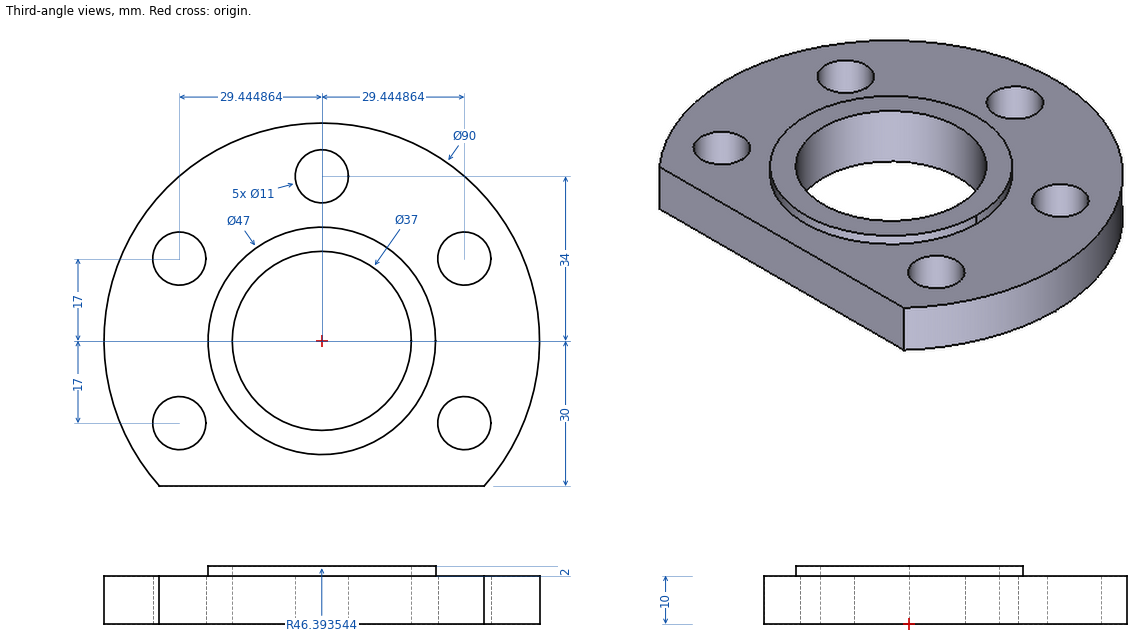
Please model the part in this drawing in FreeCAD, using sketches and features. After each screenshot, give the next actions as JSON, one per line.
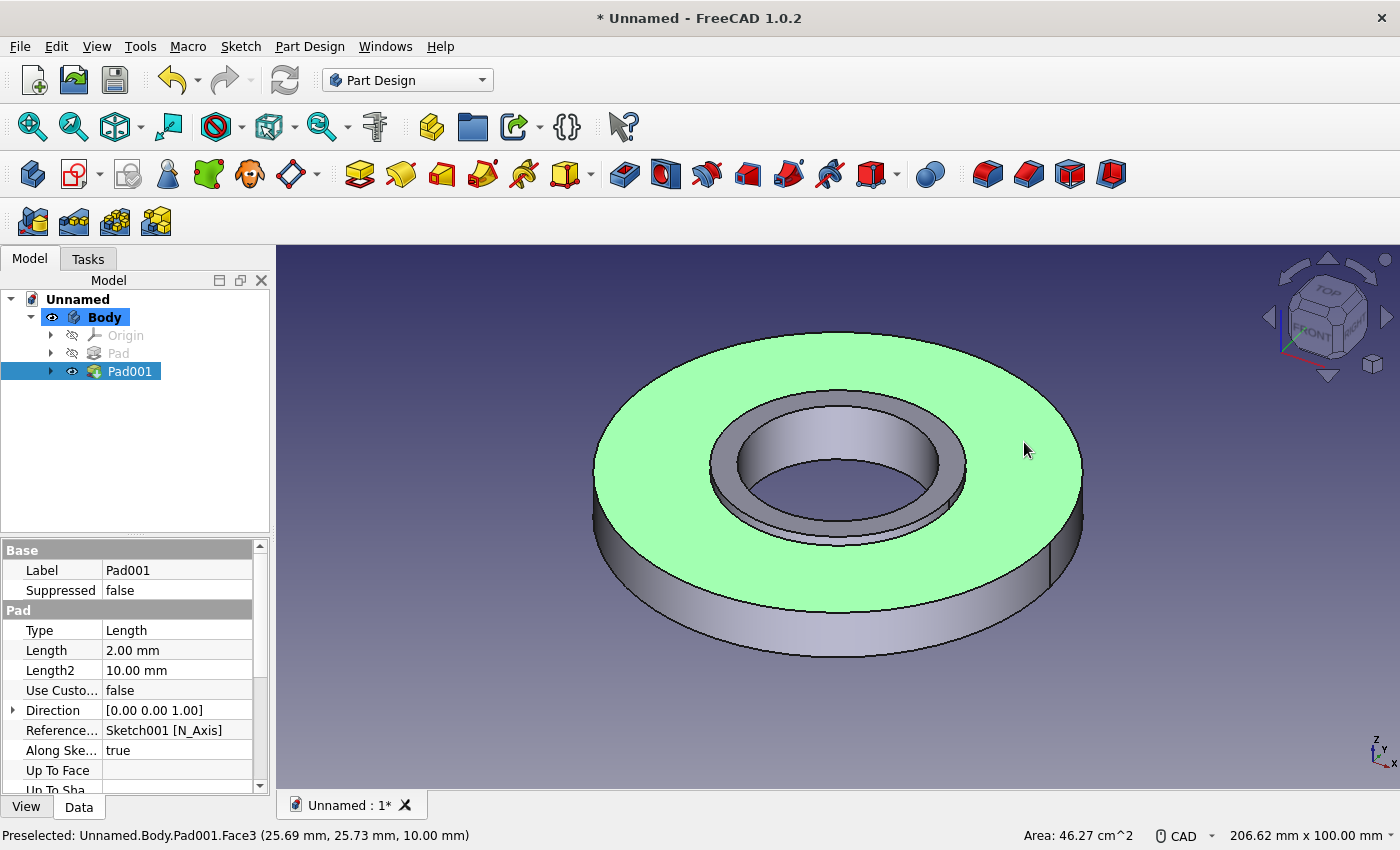
{"action": "left_click", "coordinate": [74, 174]}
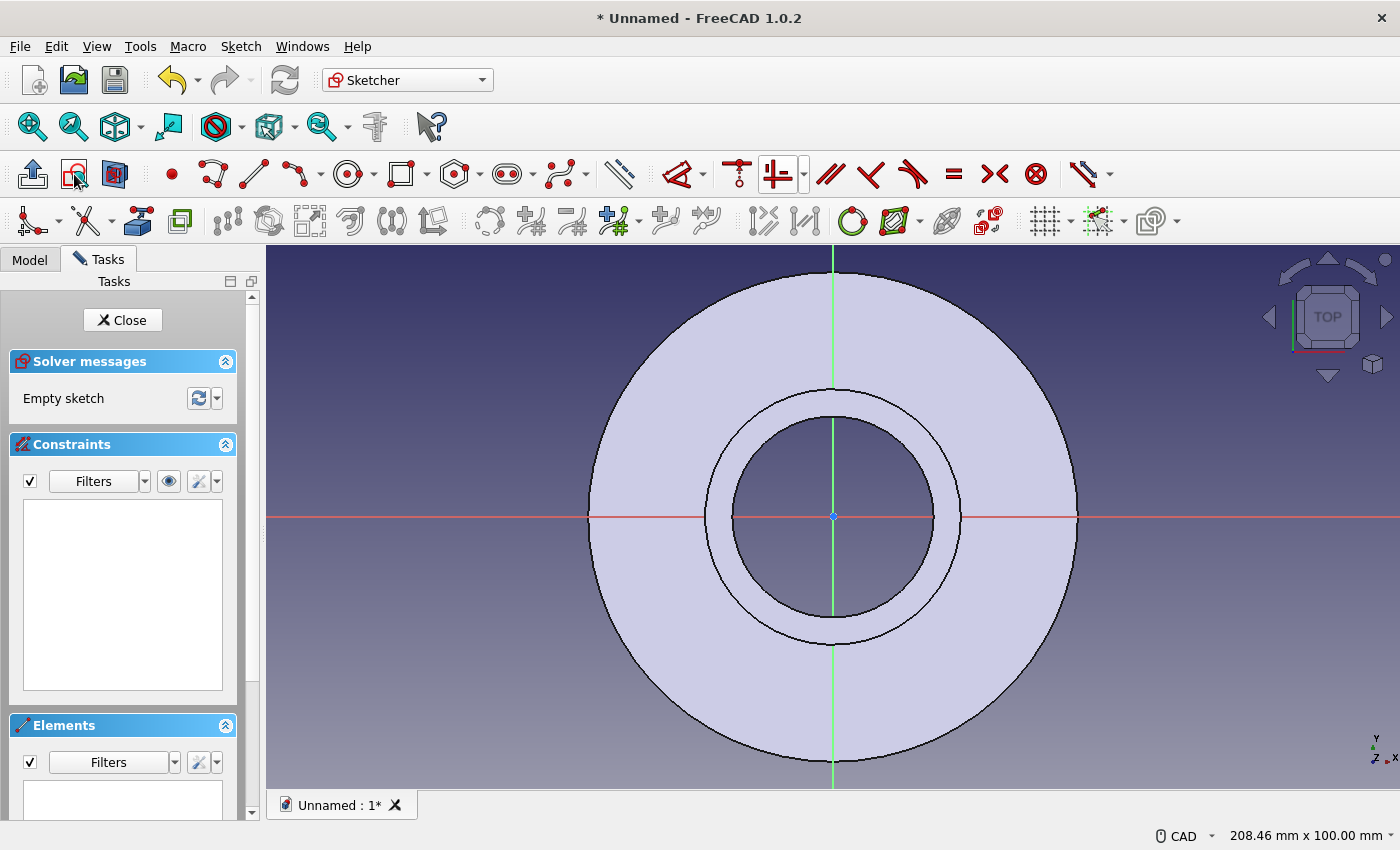
{"action": "left_click", "coordinate": [115, 174]}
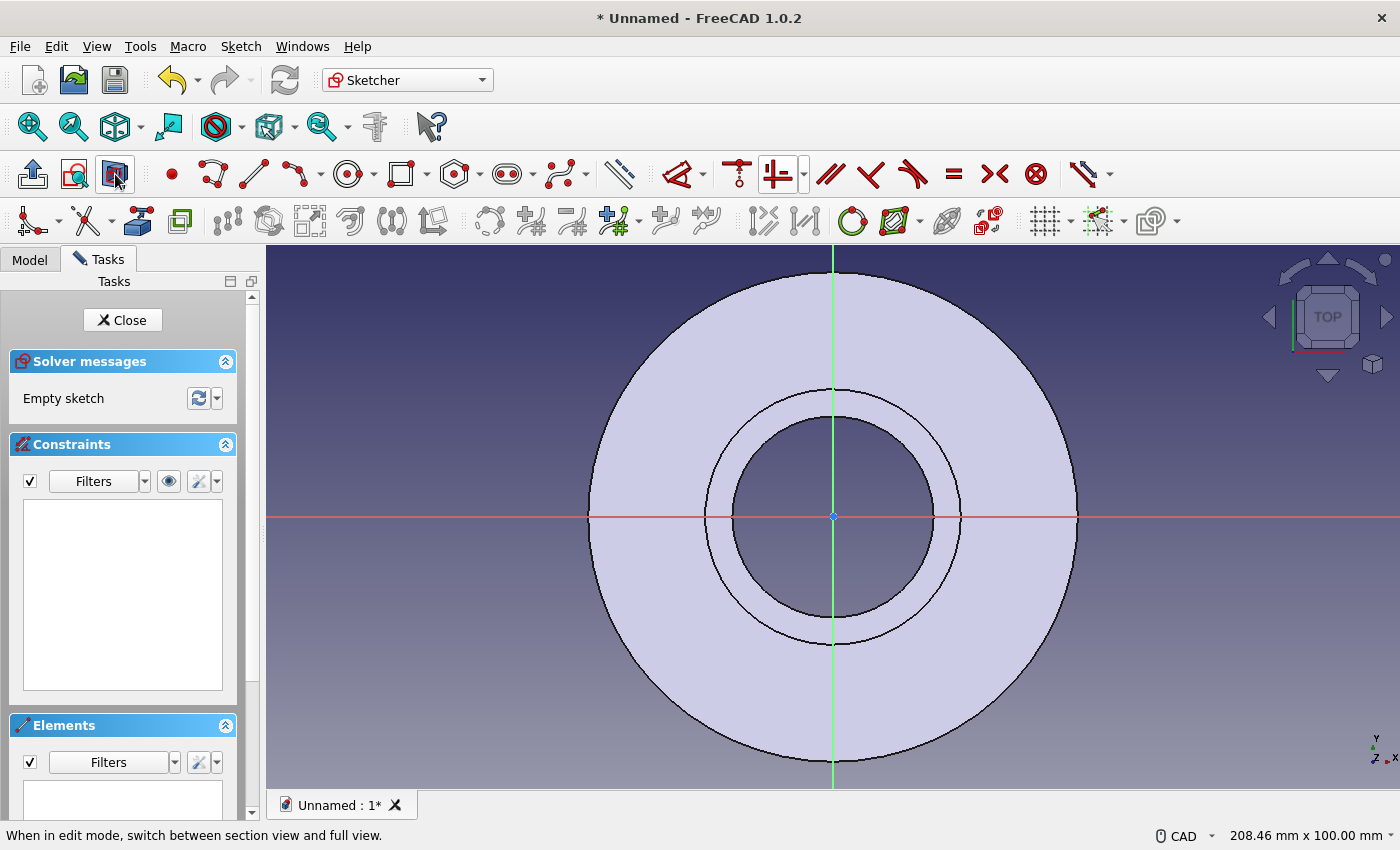
{"action": "left_click", "coordinate": [348, 174]}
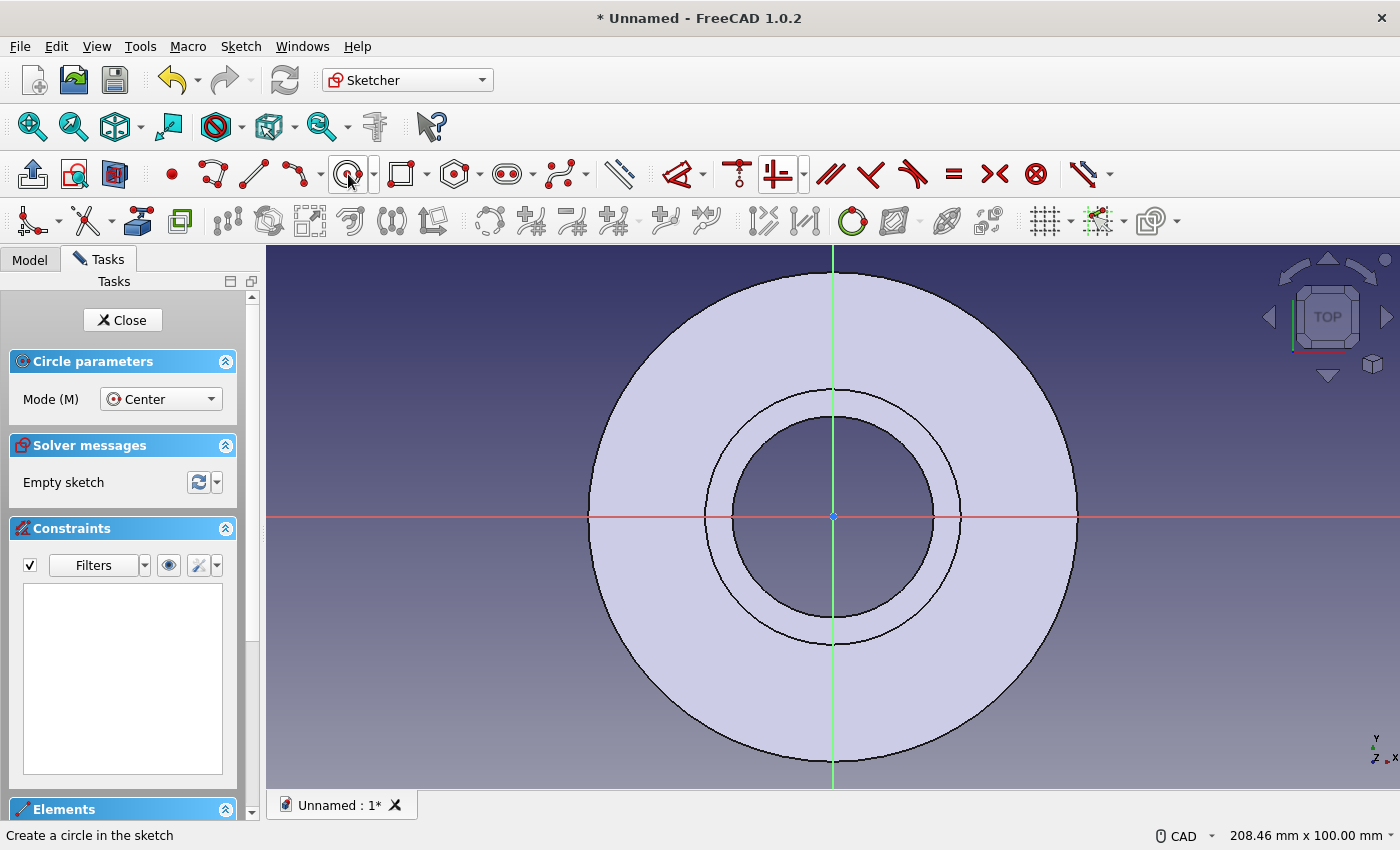
{"action": "left_click", "coordinate": [833, 332]}
{"action": "left_click", "coordinate": [854, 311]}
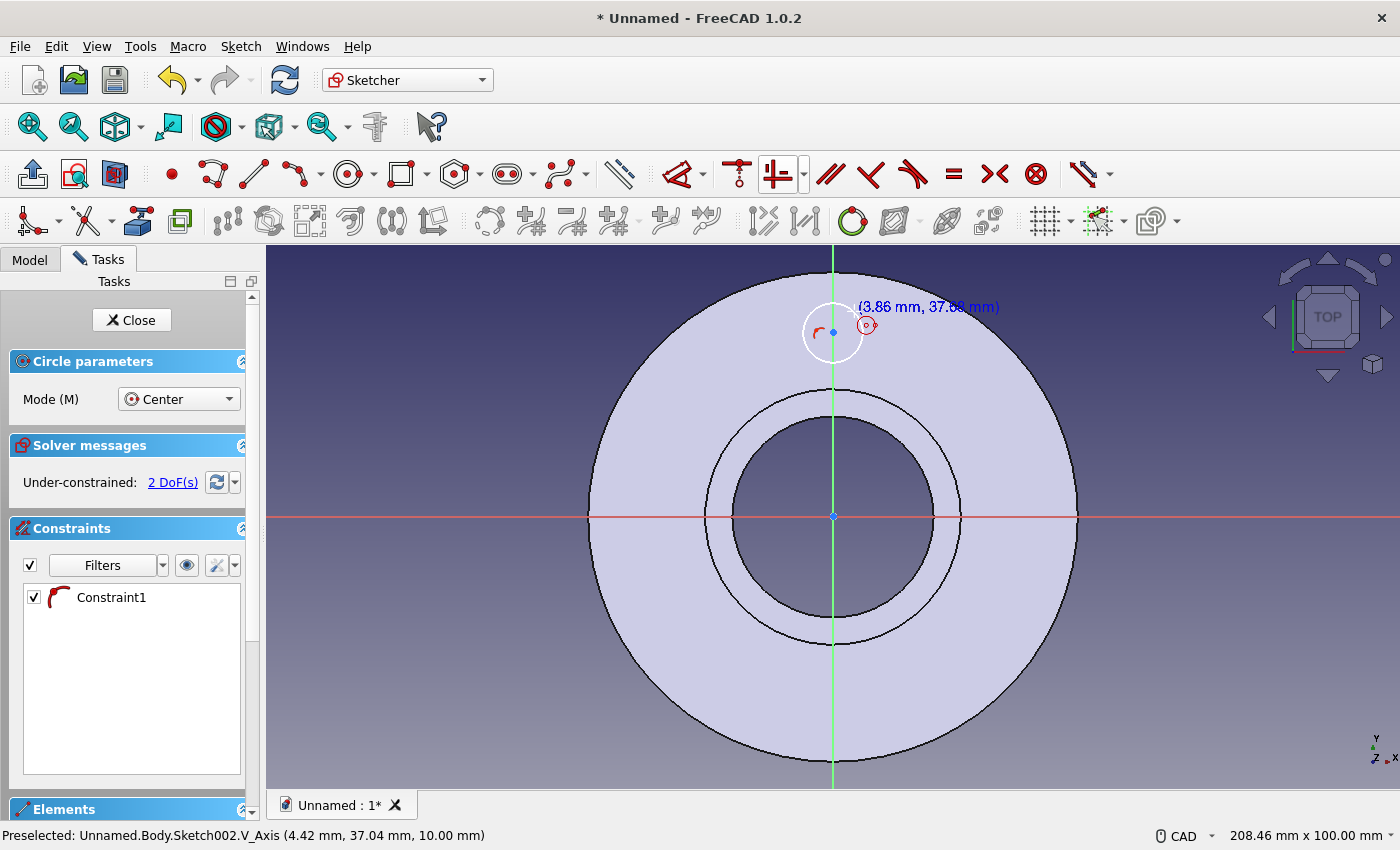
{"action": "left_click", "coordinate": [673, 425]}
{"action": "left_click", "coordinate": [694, 403]}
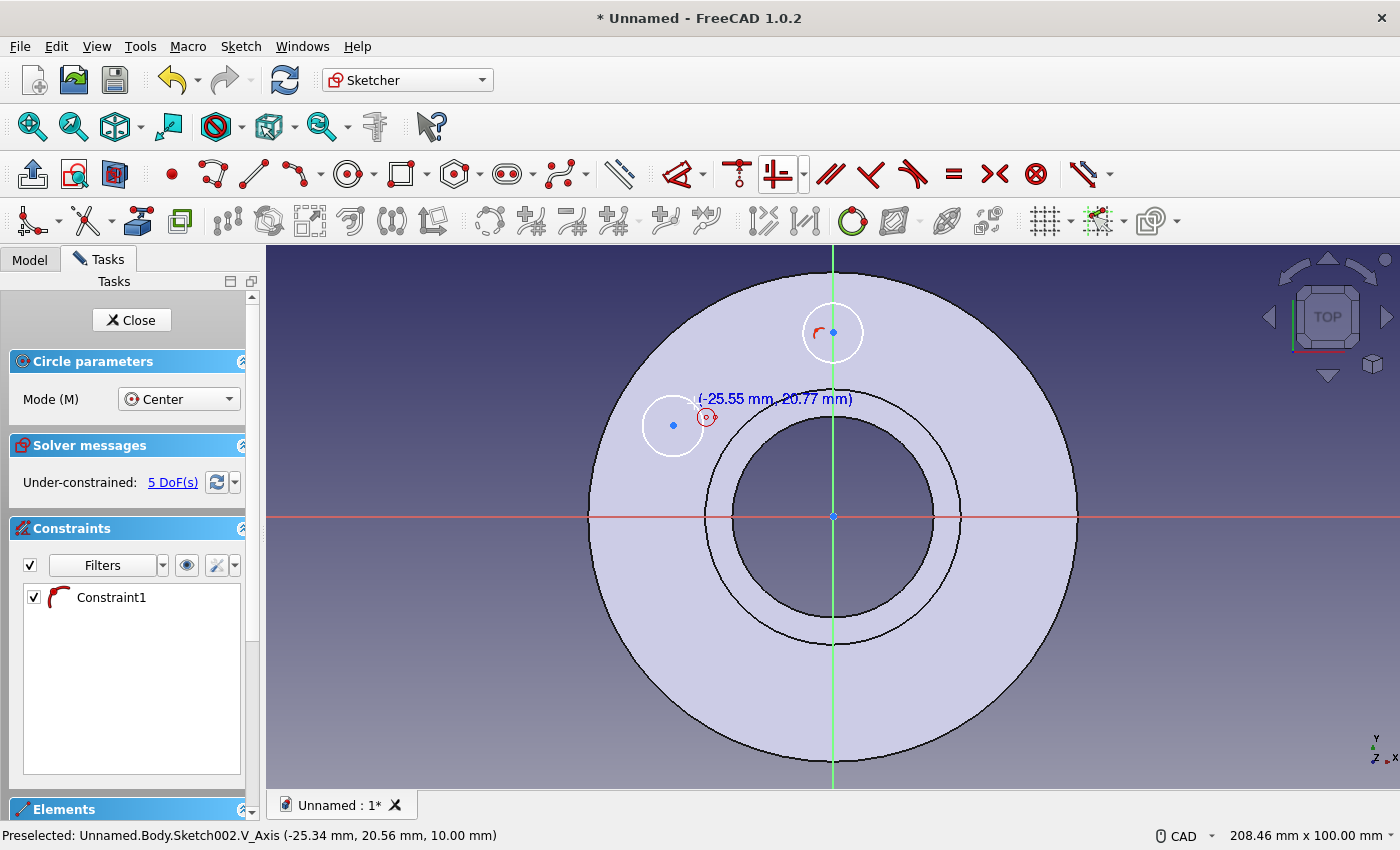
{"action": "left_click", "coordinate": [673, 609]}
{"action": "left_click", "coordinate": [694, 588]}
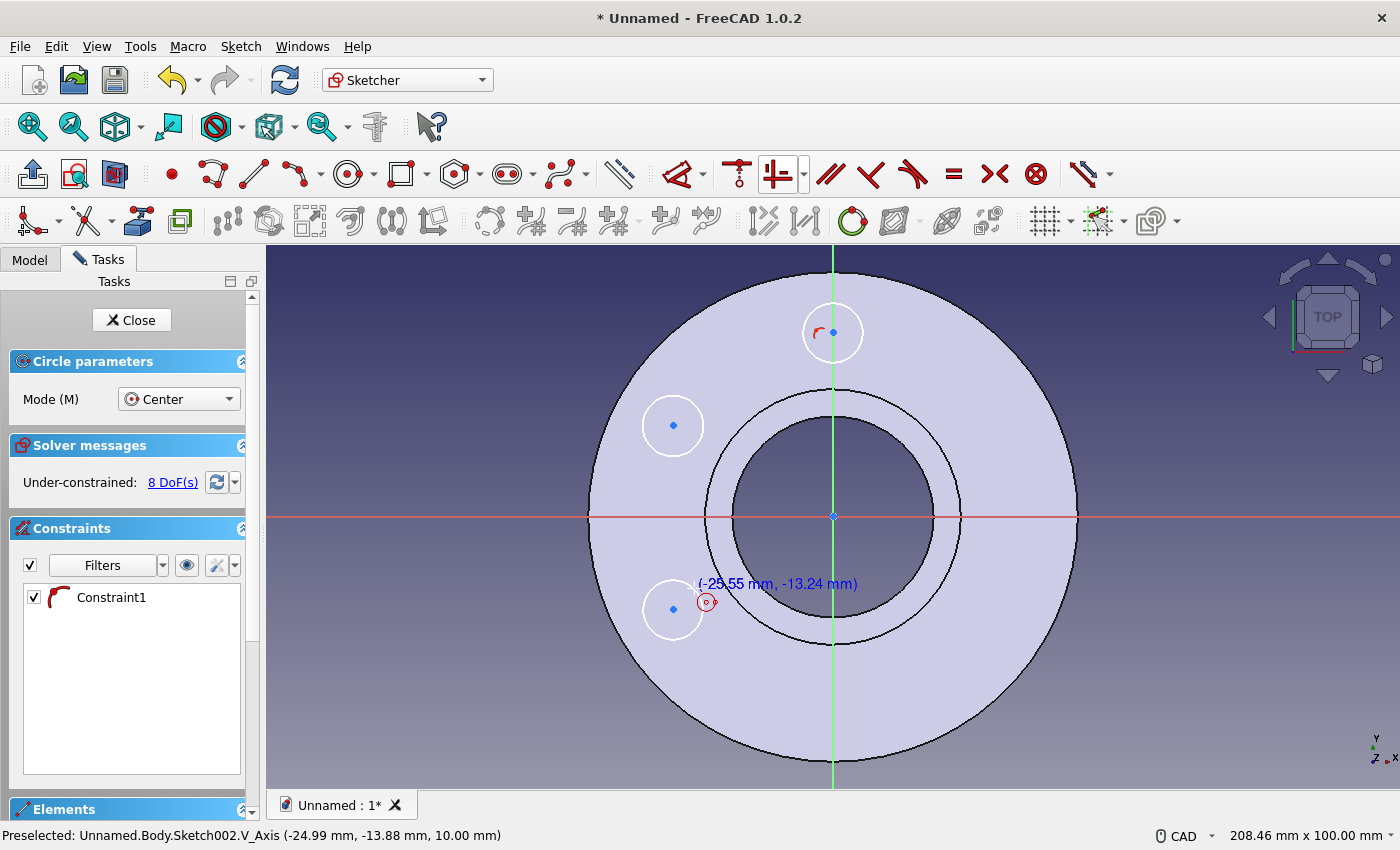
{"action": "left_click", "coordinate": [993, 425]}
{"action": "left_click", "coordinate": [1014, 403]}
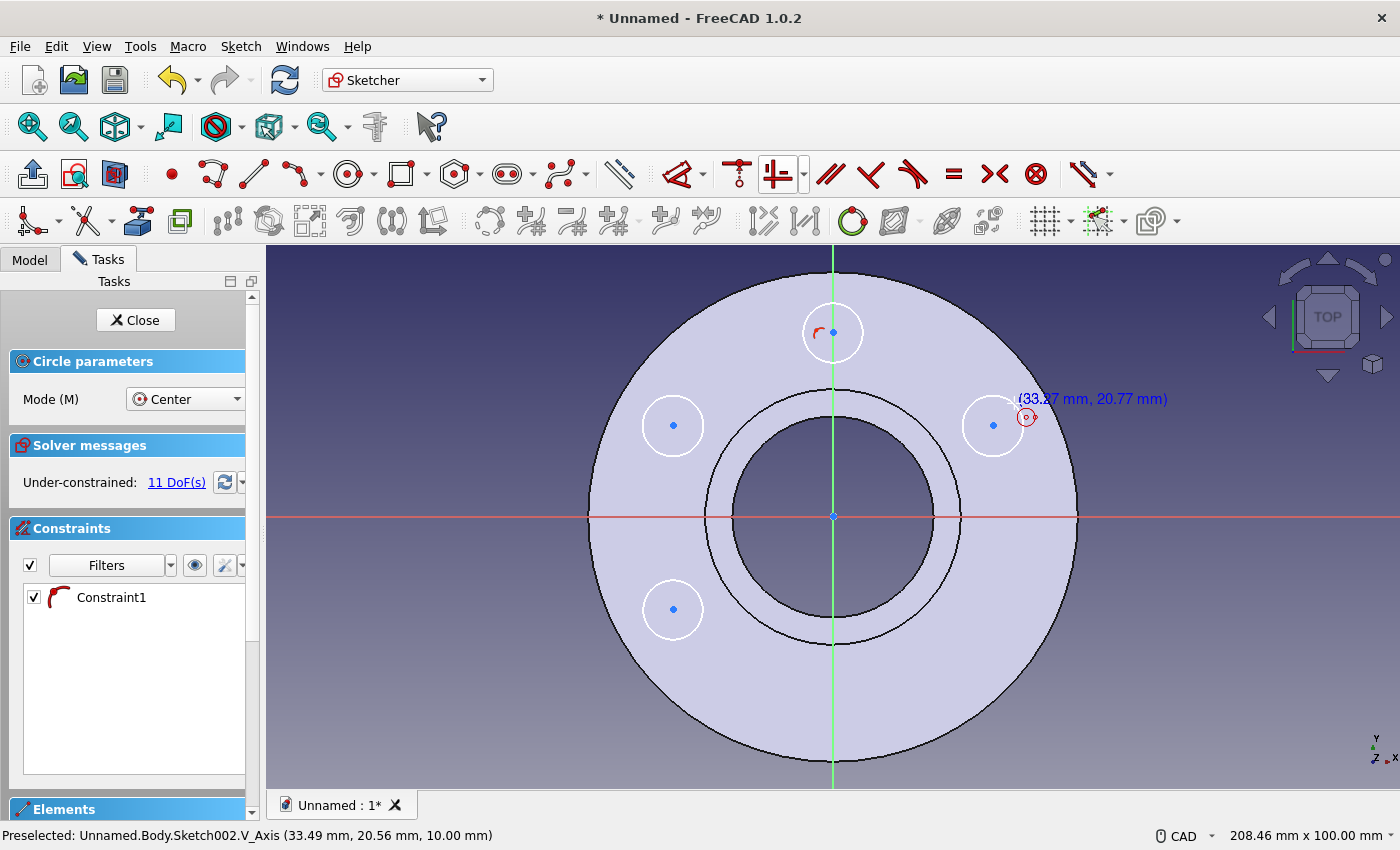
{"action": "left_click", "coordinate": [993, 609]}
{"action": "left_click", "coordinate": [1014, 588]}
{"action": "key", "text": "Escape"}